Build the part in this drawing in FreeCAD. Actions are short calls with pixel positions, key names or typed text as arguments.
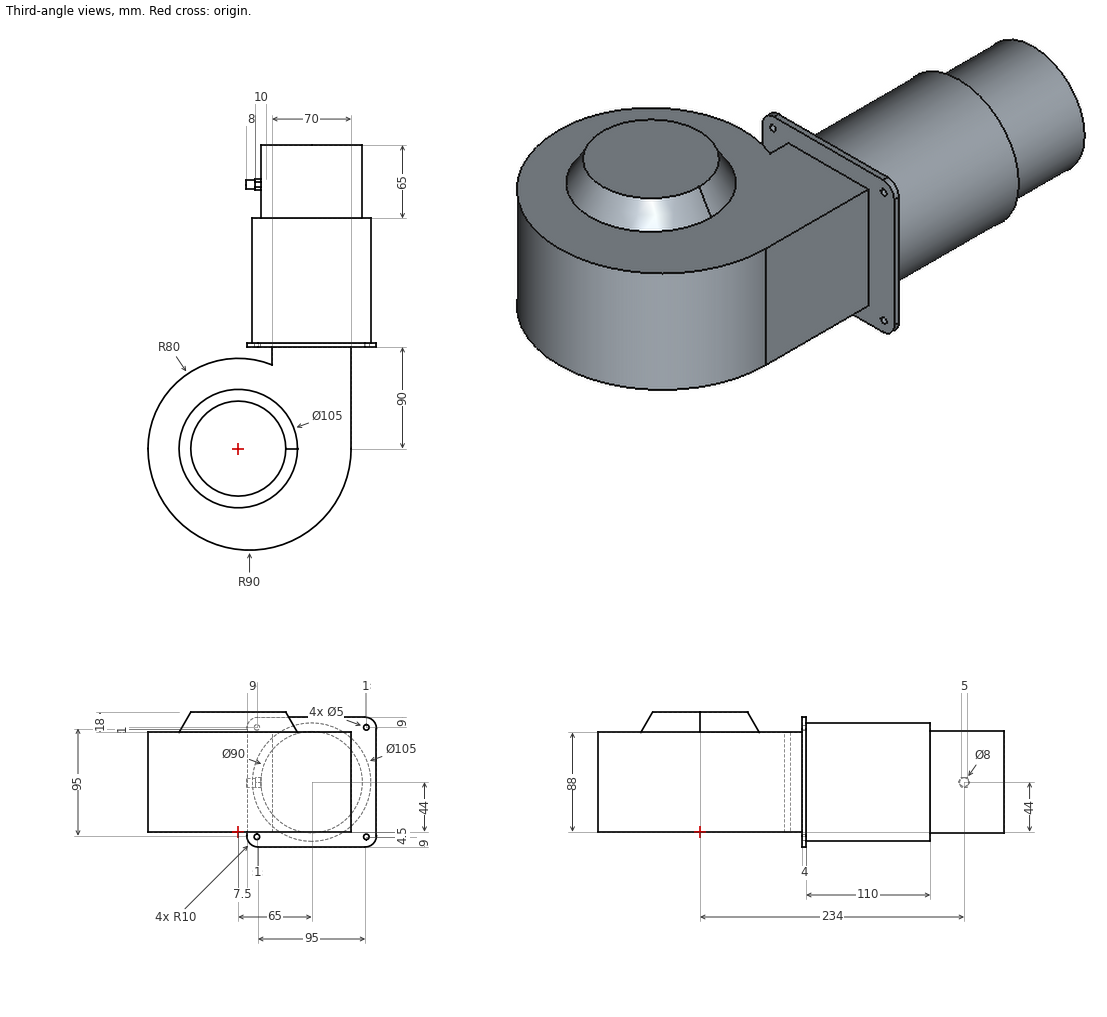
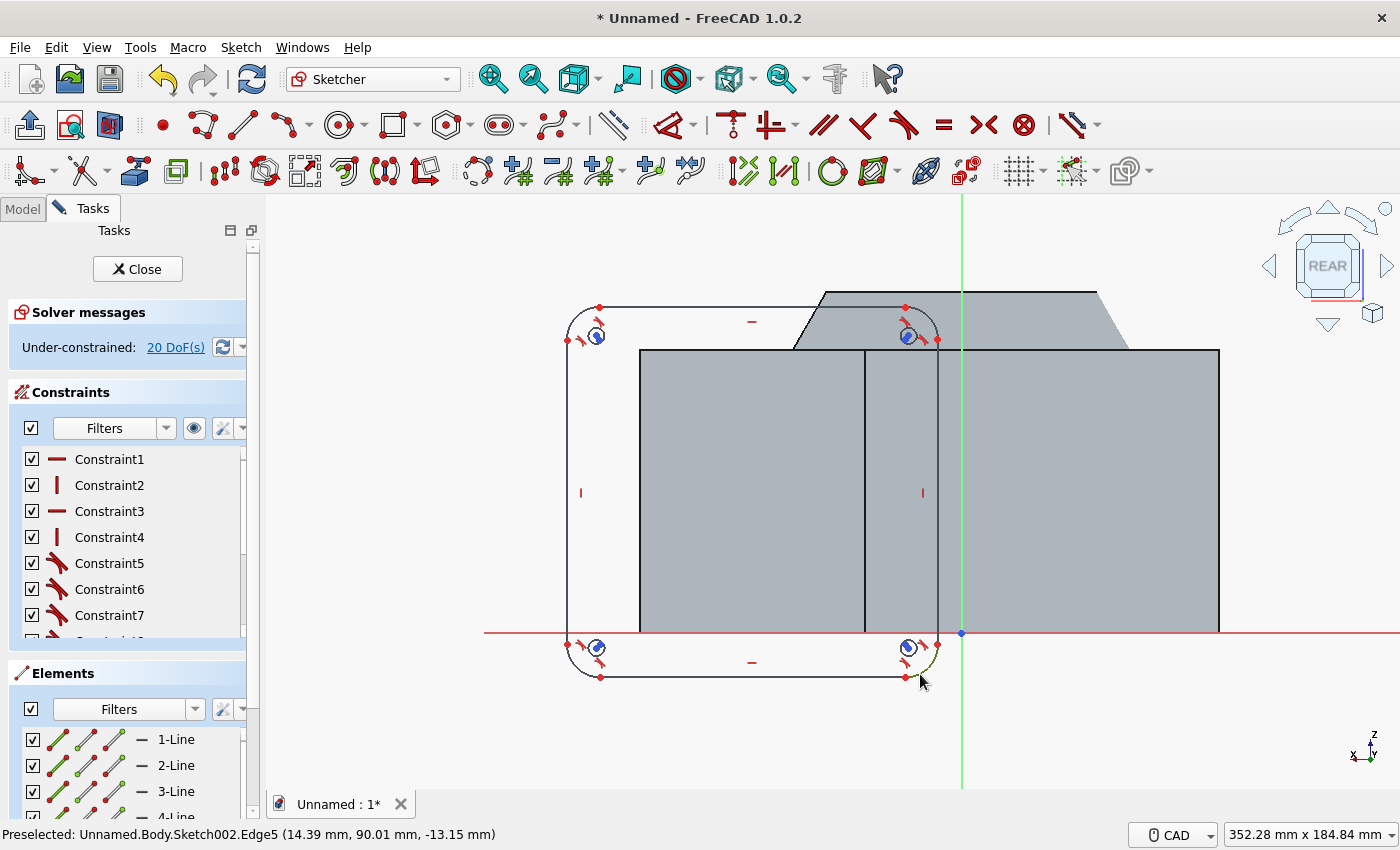
click(934, 325)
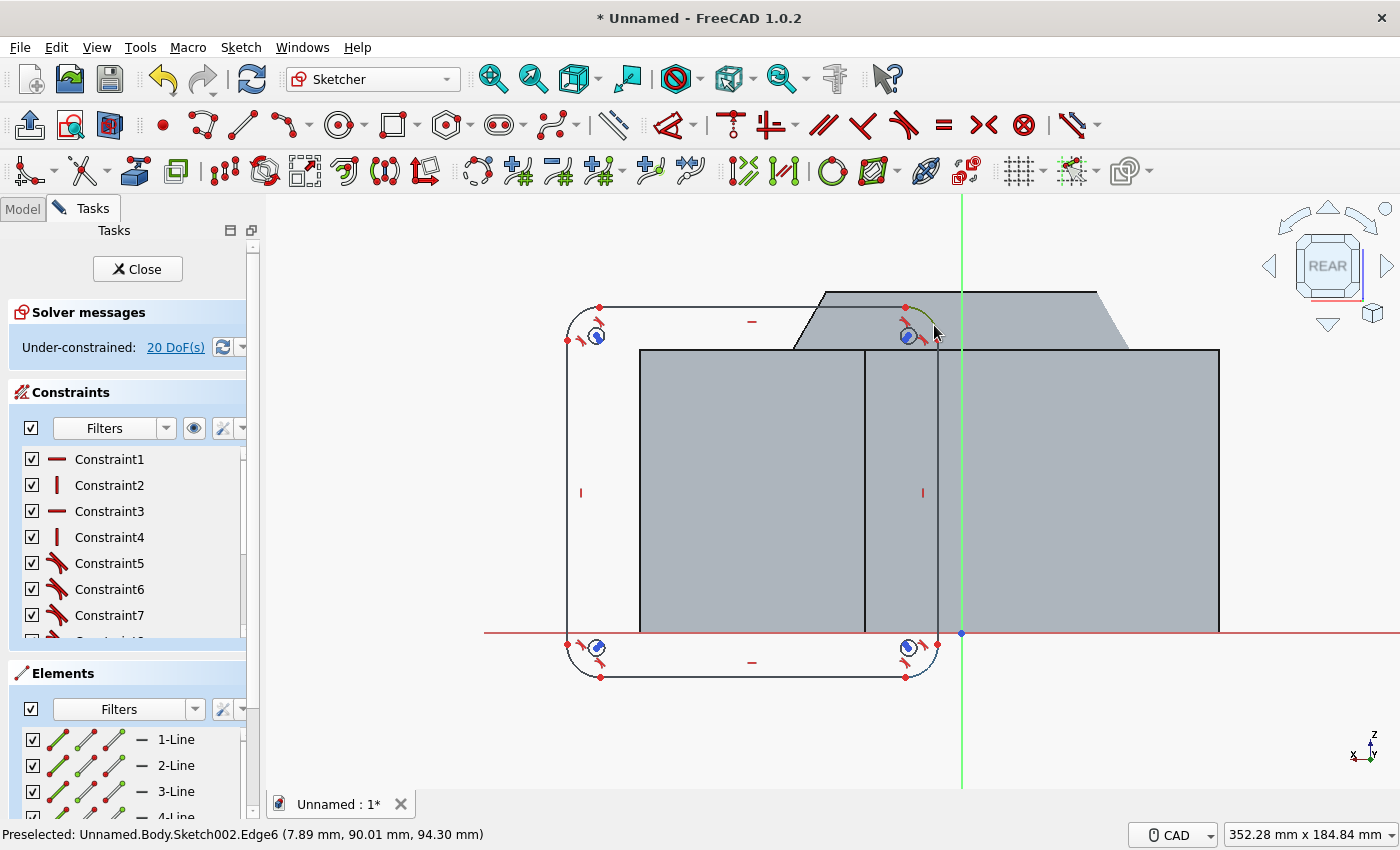
click(585, 311)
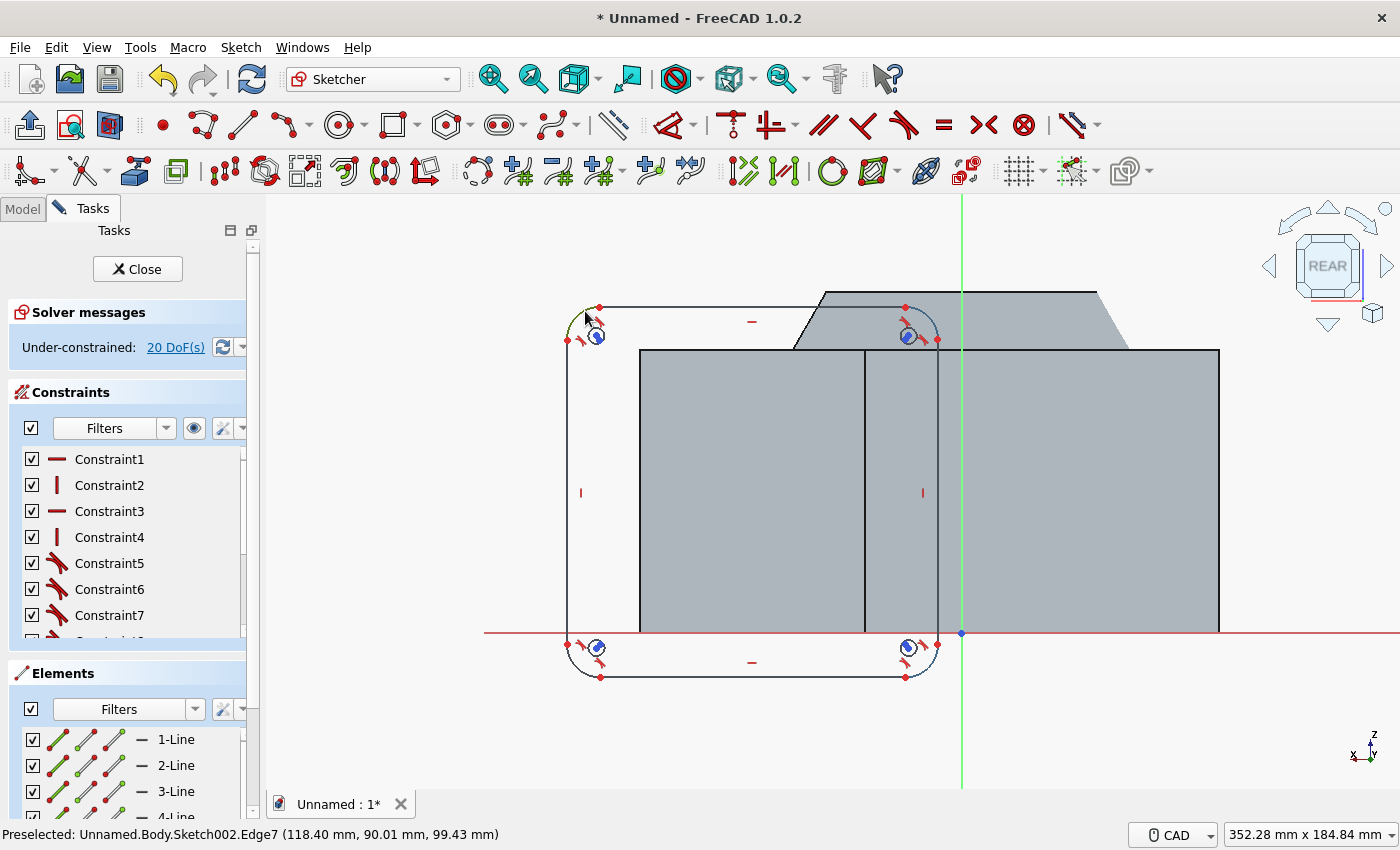
click(571, 659)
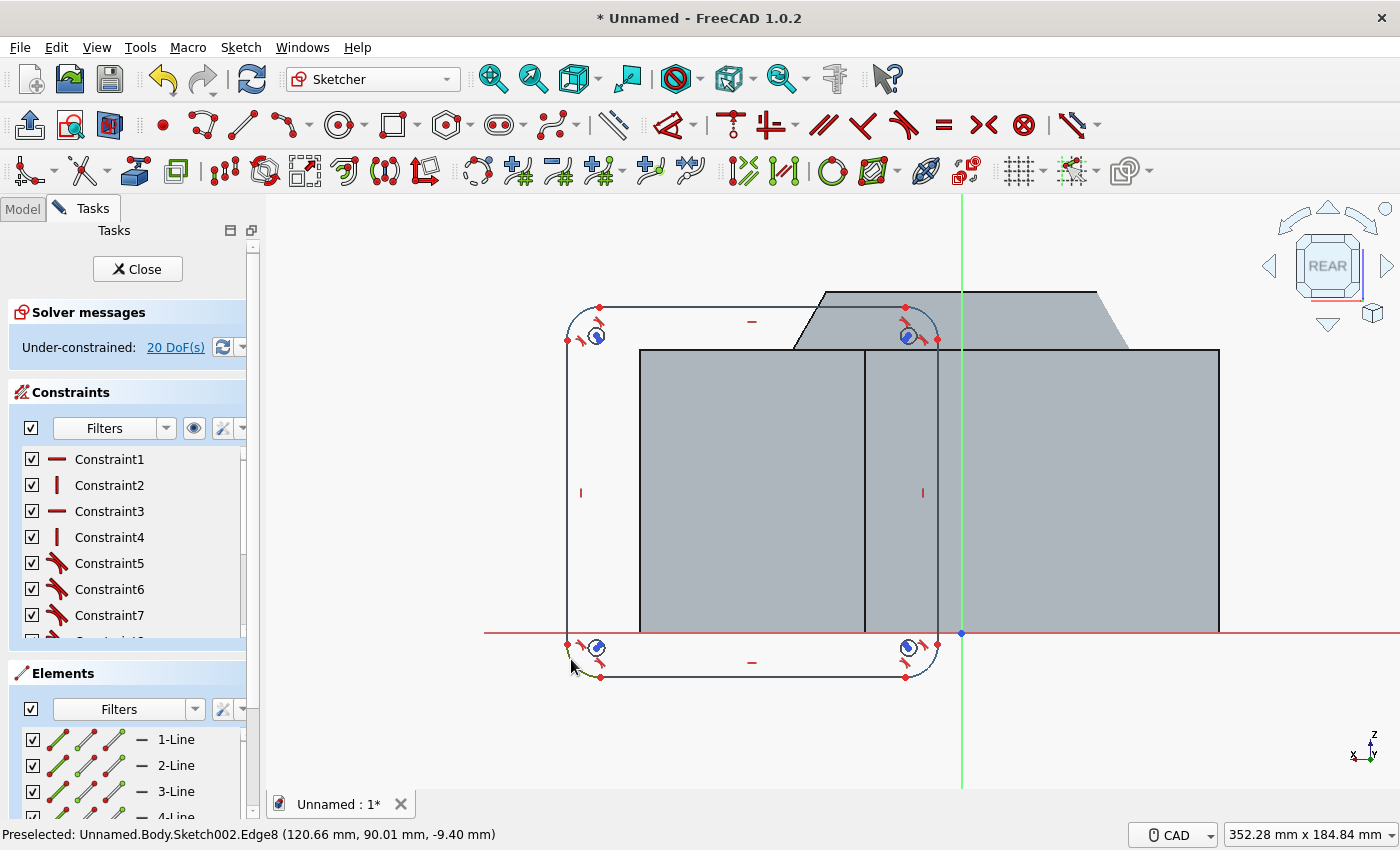
click(944, 126)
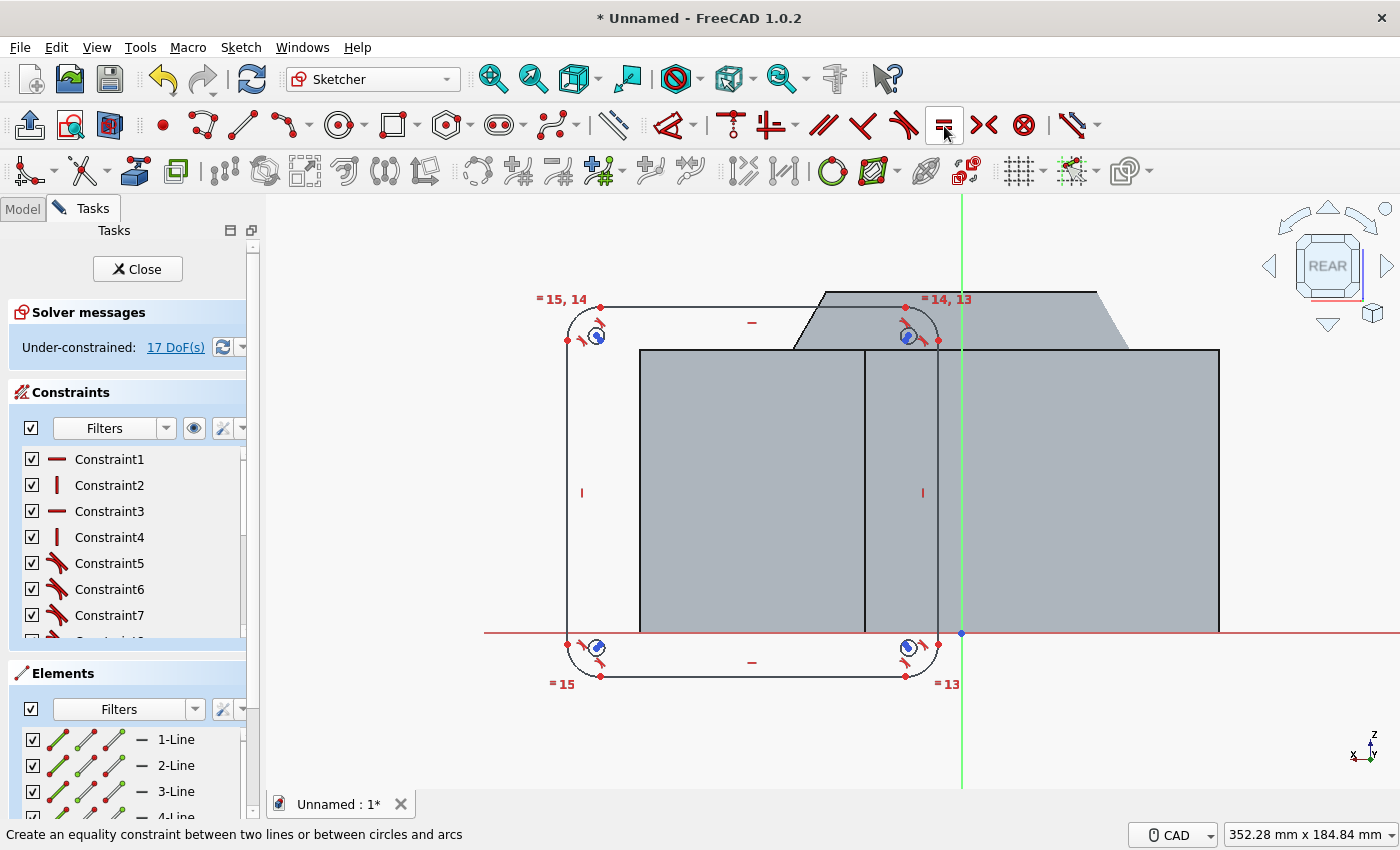
scroll(597, 328, up, 3)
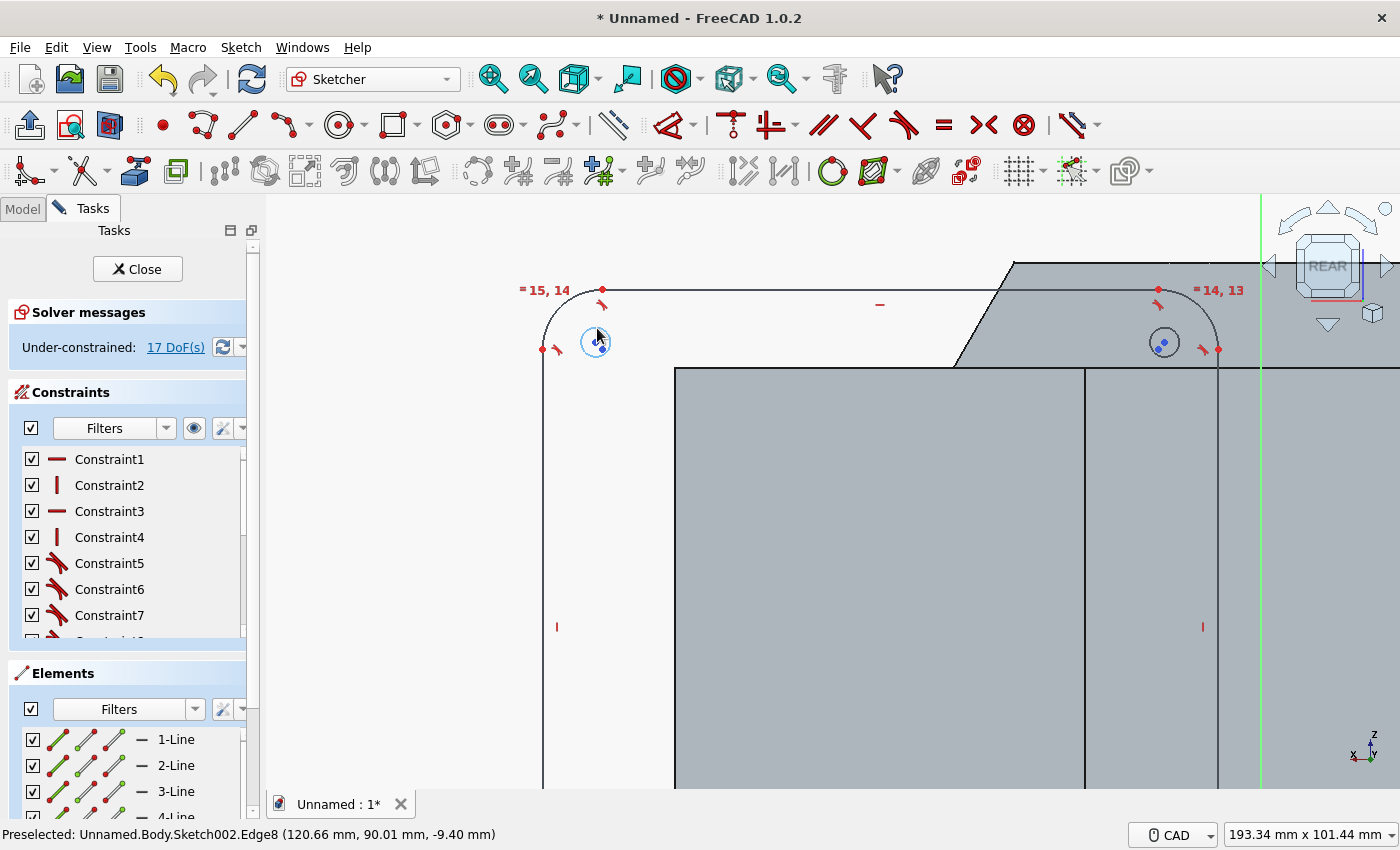
click(596, 328)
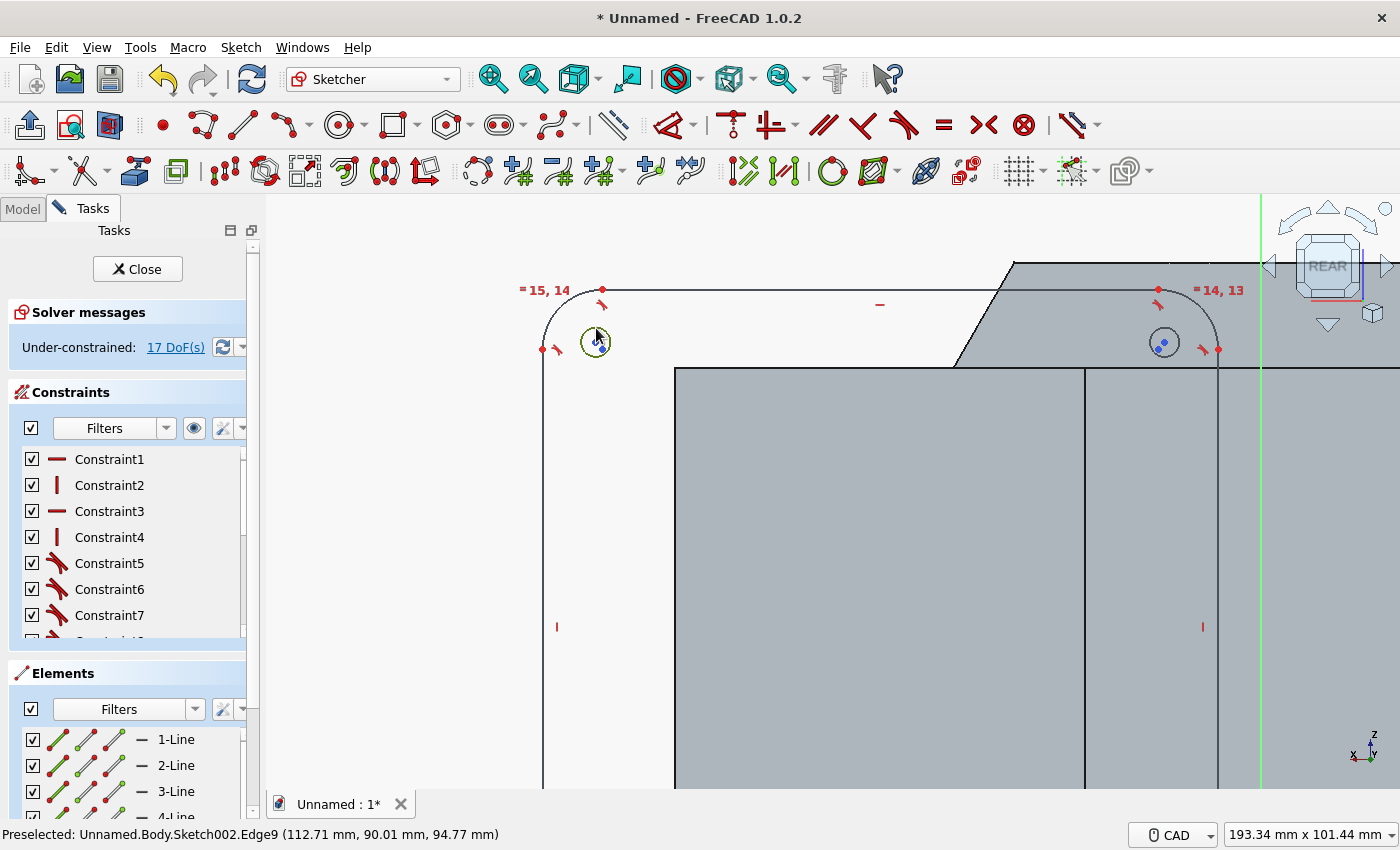
click(1175, 332)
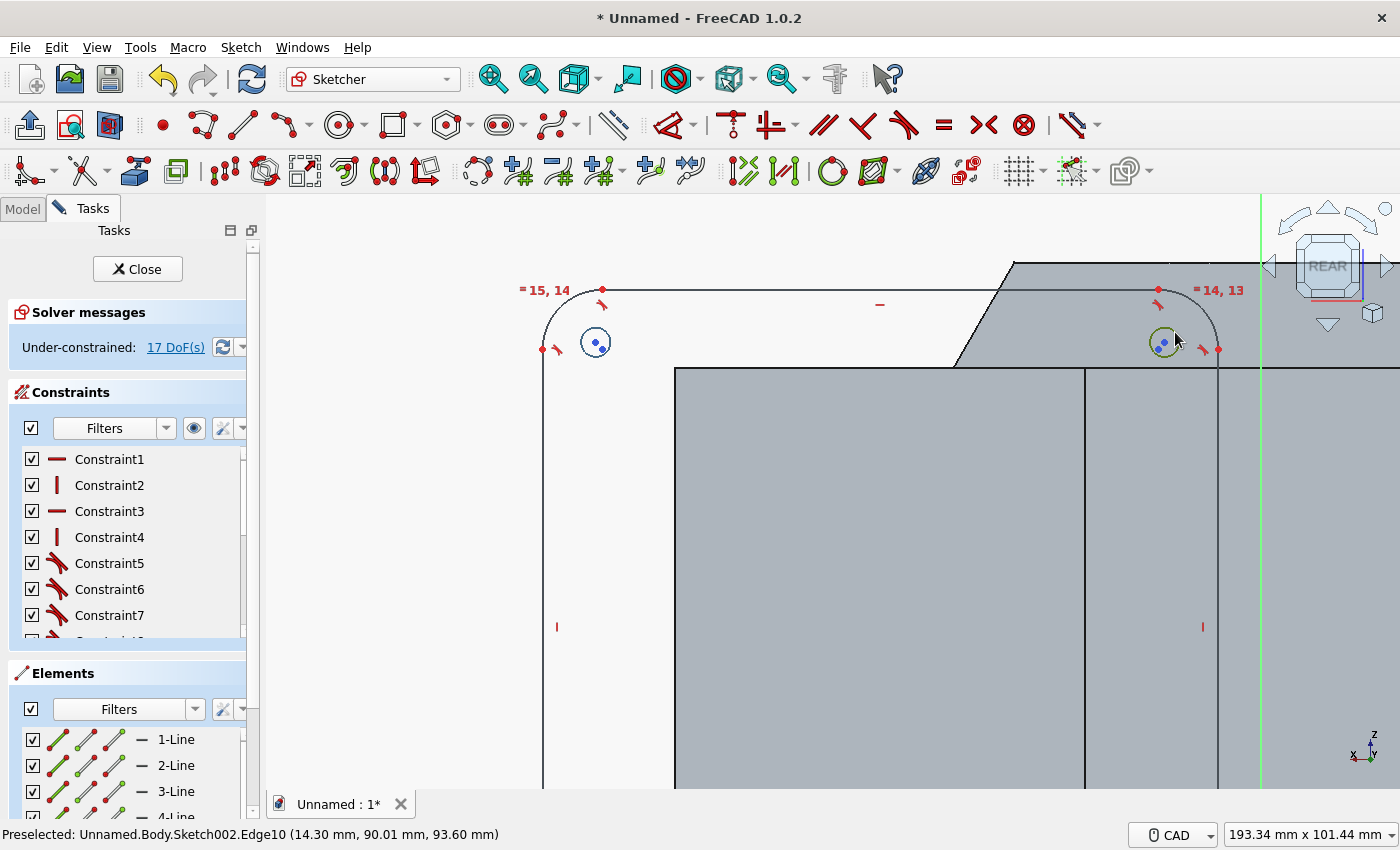
scroll(597, 328, down, 3)